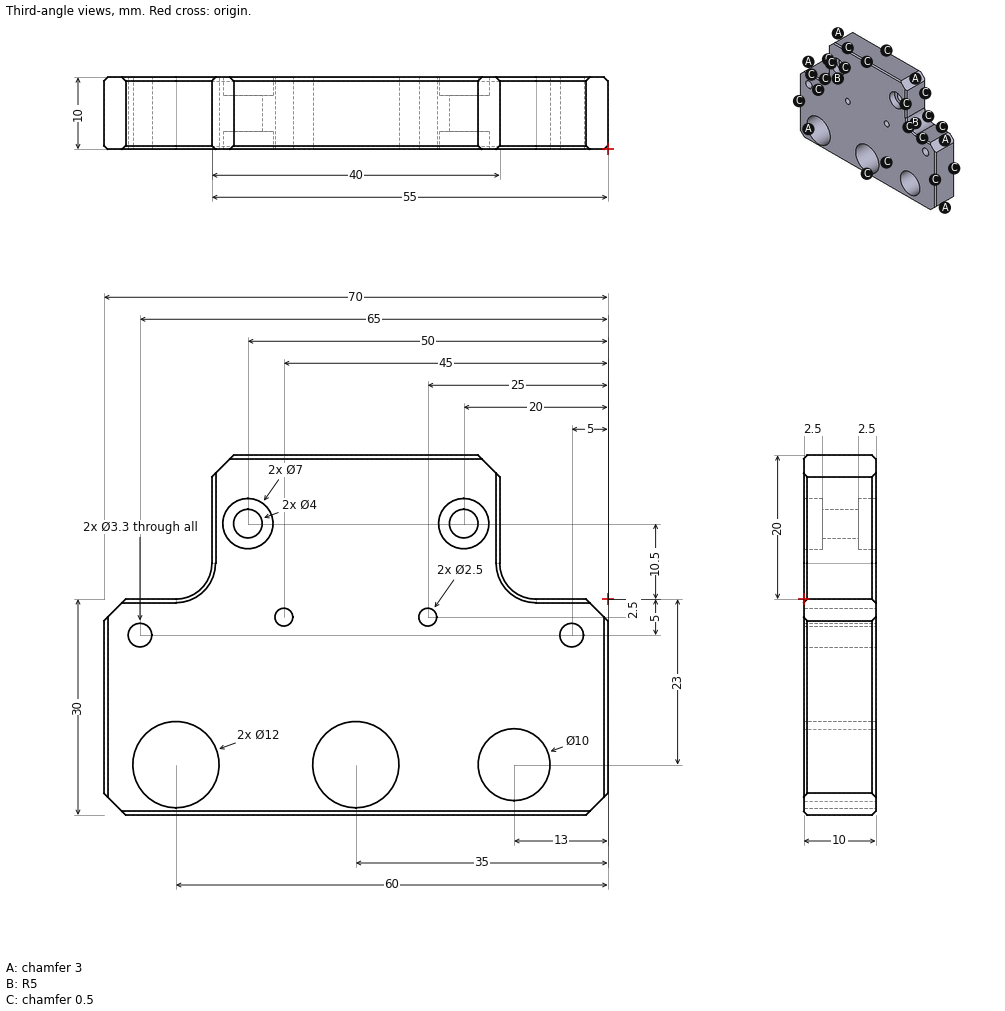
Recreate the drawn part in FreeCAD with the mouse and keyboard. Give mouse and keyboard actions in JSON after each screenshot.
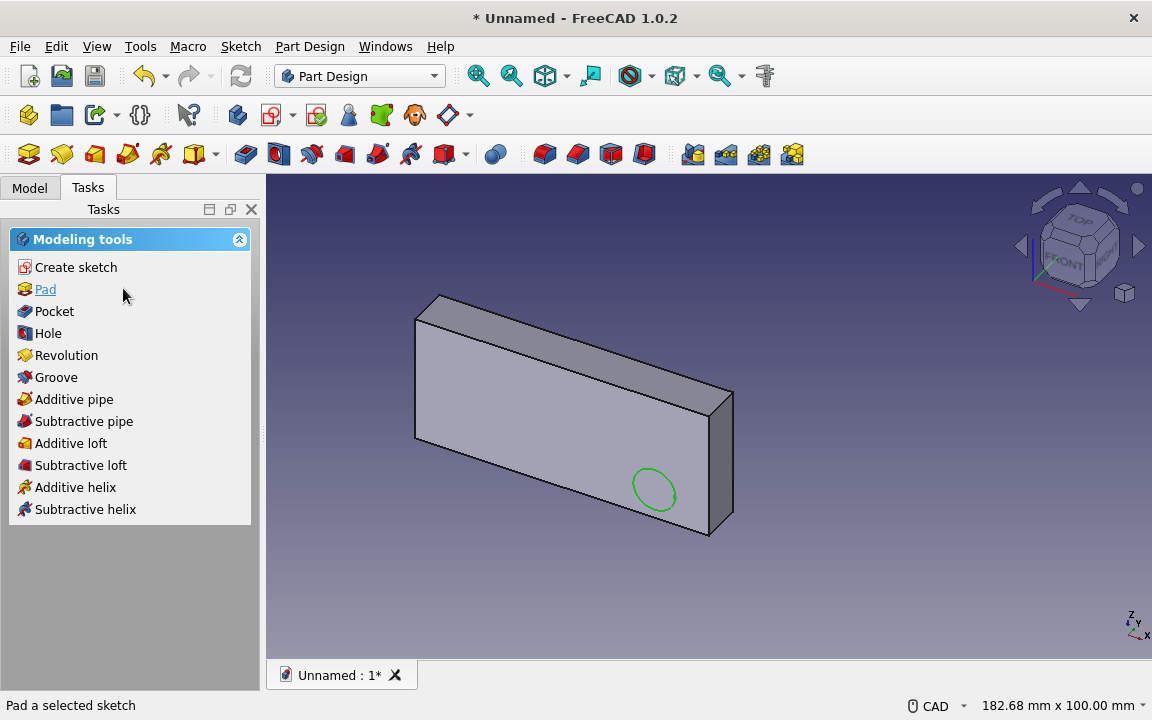
{"action": "left_click", "coordinate": [246, 154]}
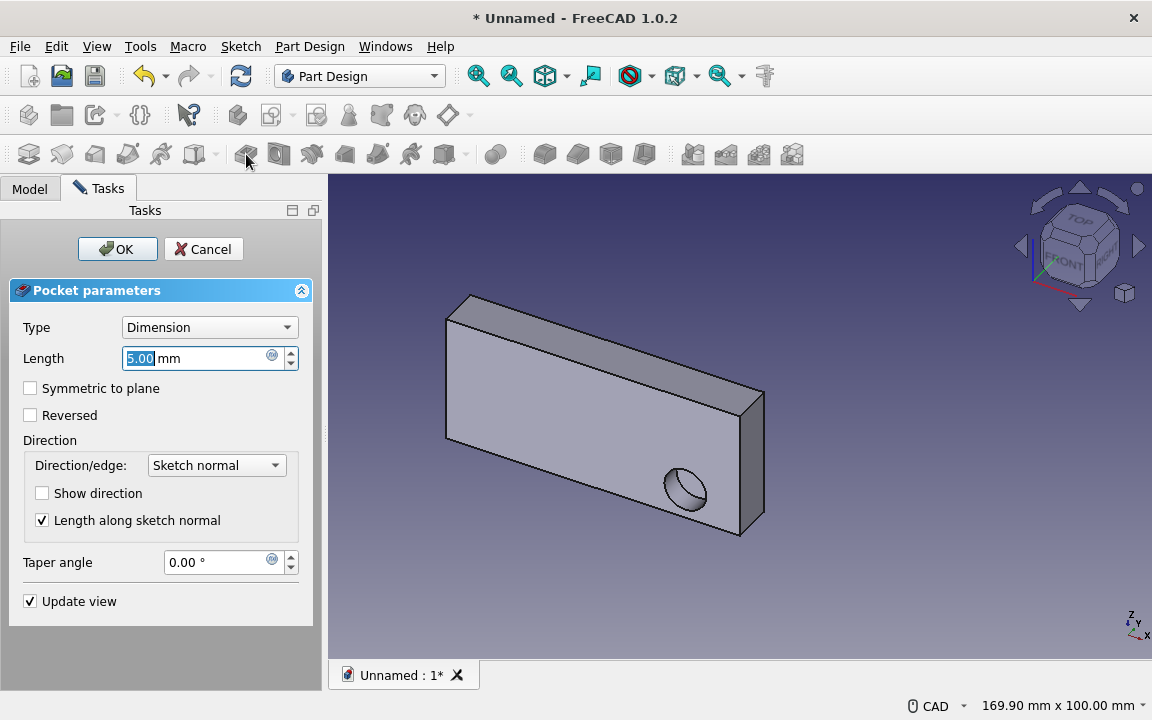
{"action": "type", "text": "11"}
{"action": "key", "text": "Tab"}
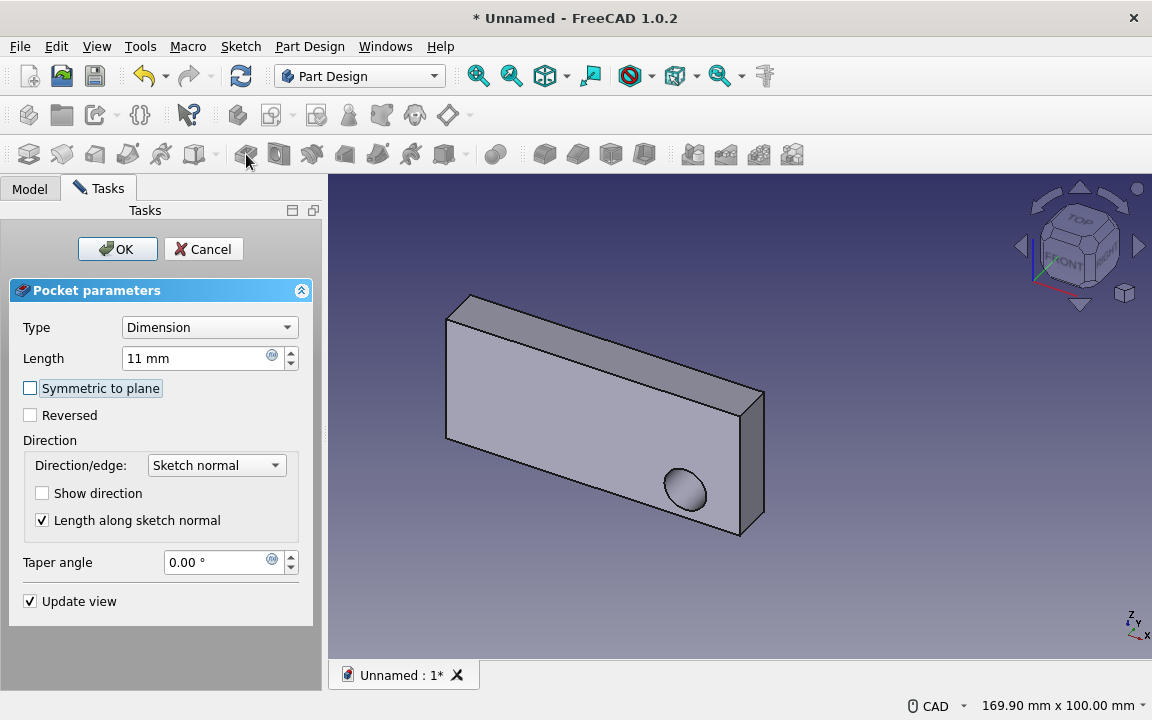
{"action": "left_click", "coordinate": [118, 249]}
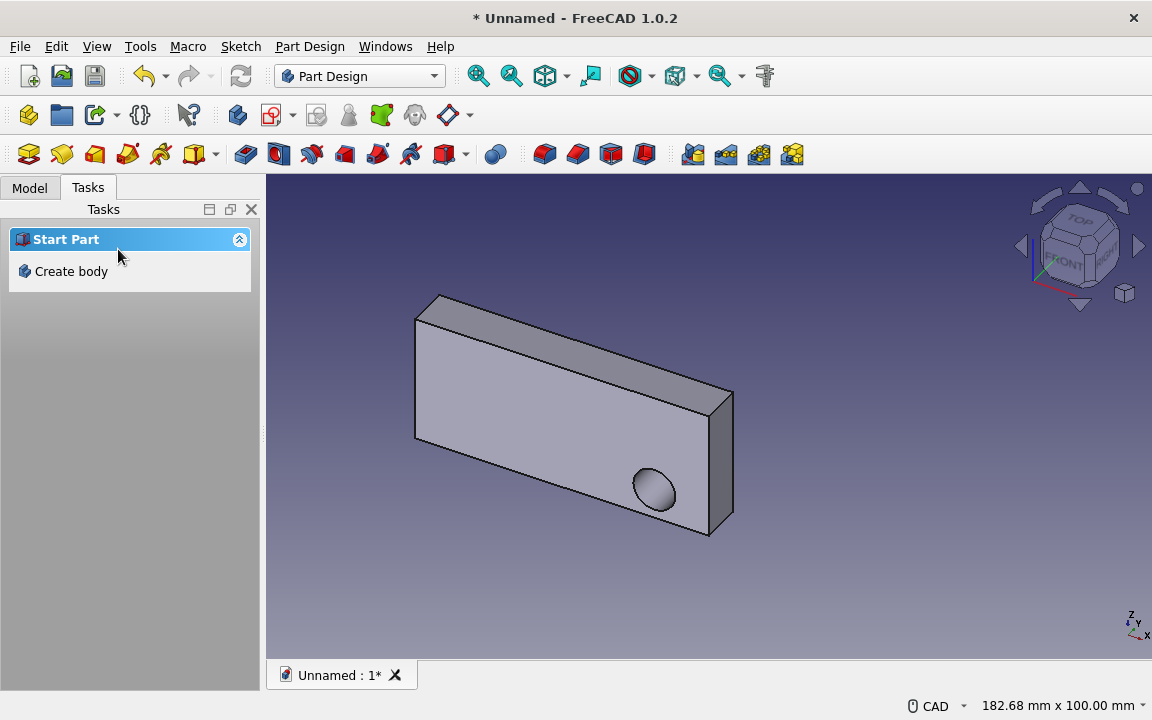
{"action": "left_click", "coordinate": [270, 116]}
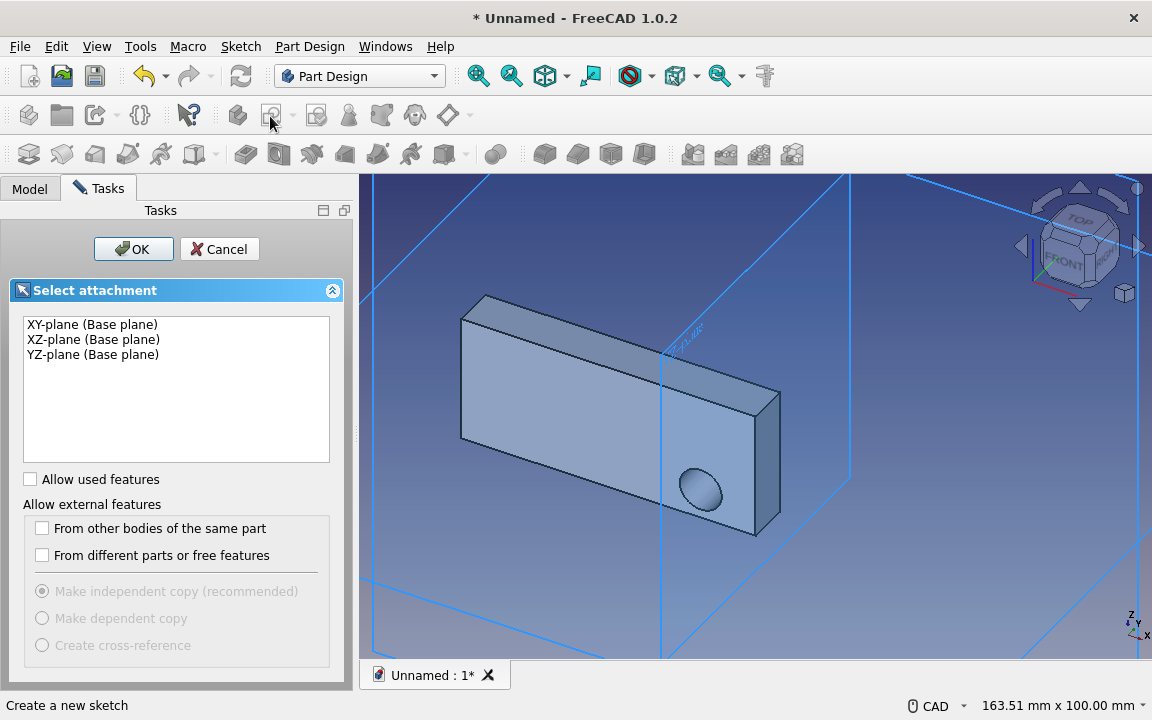
{"action": "left_click", "coordinate": [84, 340]}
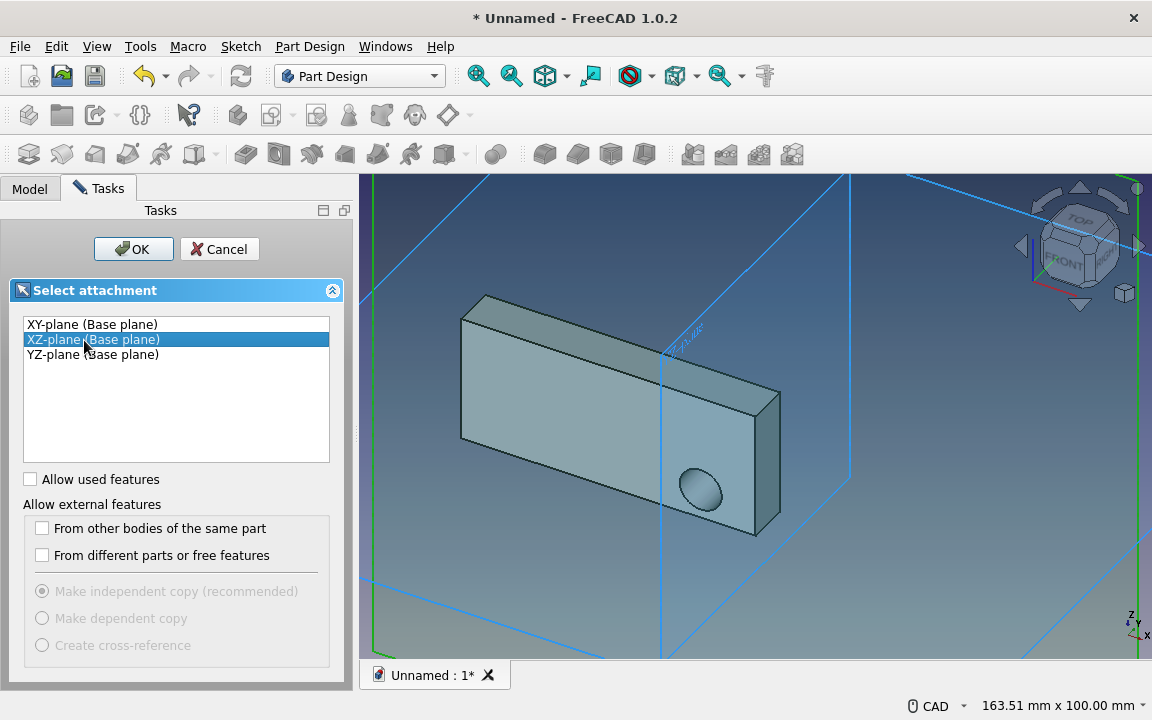
{"action": "left_click", "coordinate": [134, 249]}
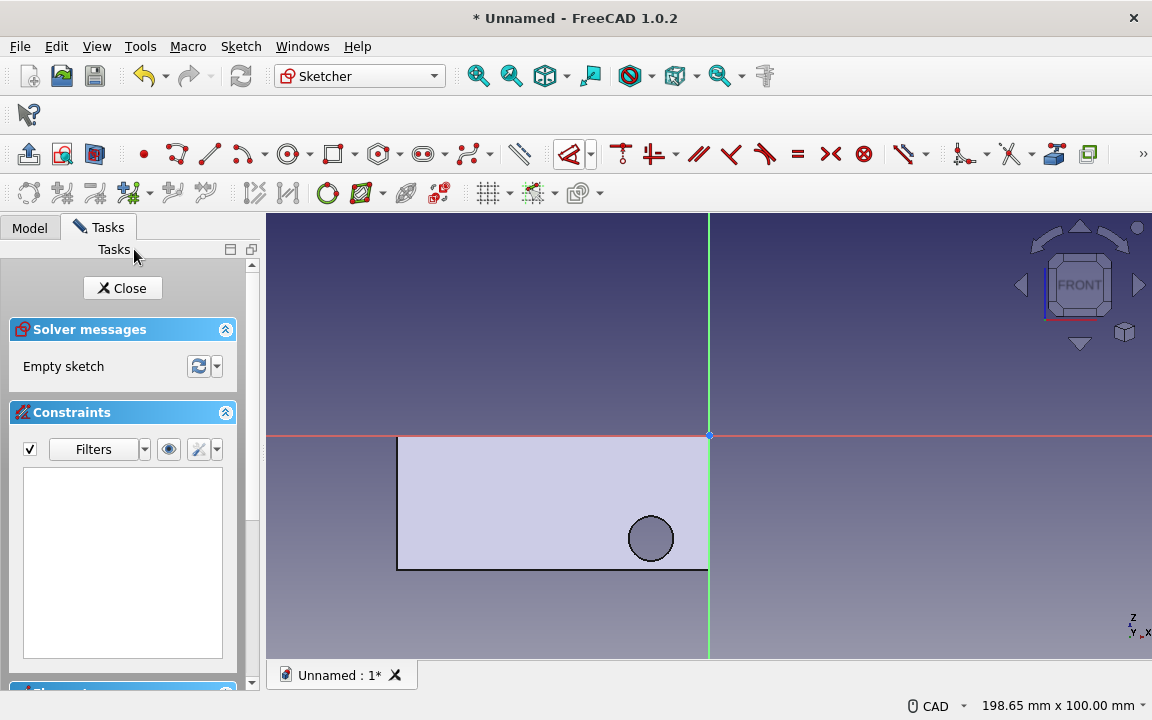
{"action": "scroll", "coordinate": [466, 579], "scroll_direction": "up", "scroll_amount": 3}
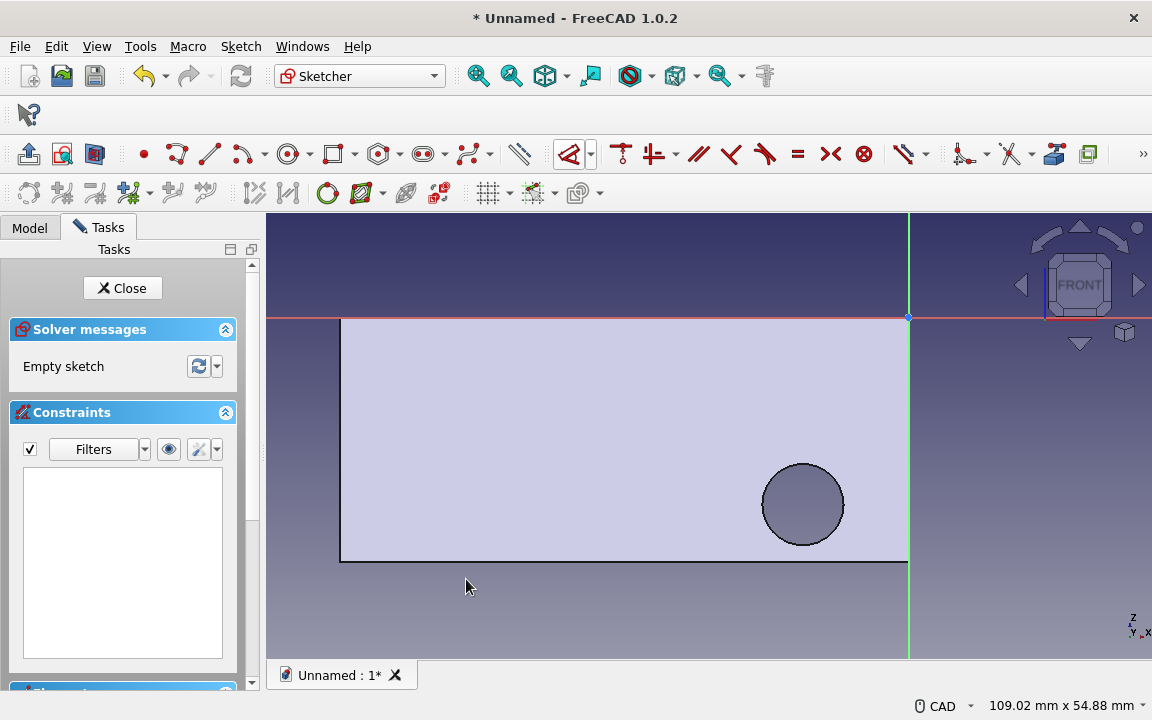
{"action": "left_click", "coordinate": [288, 154]}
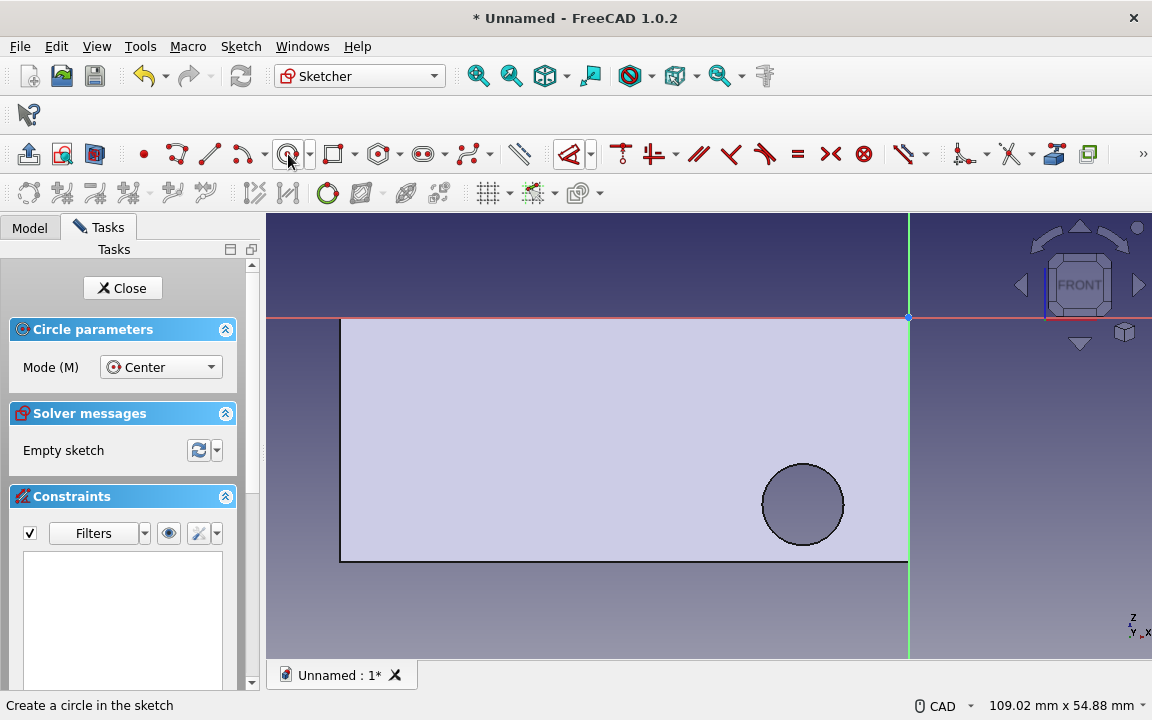
{"action": "left_click", "coordinate": [421, 505]}
{"action": "left_click", "coordinate": [455, 470]}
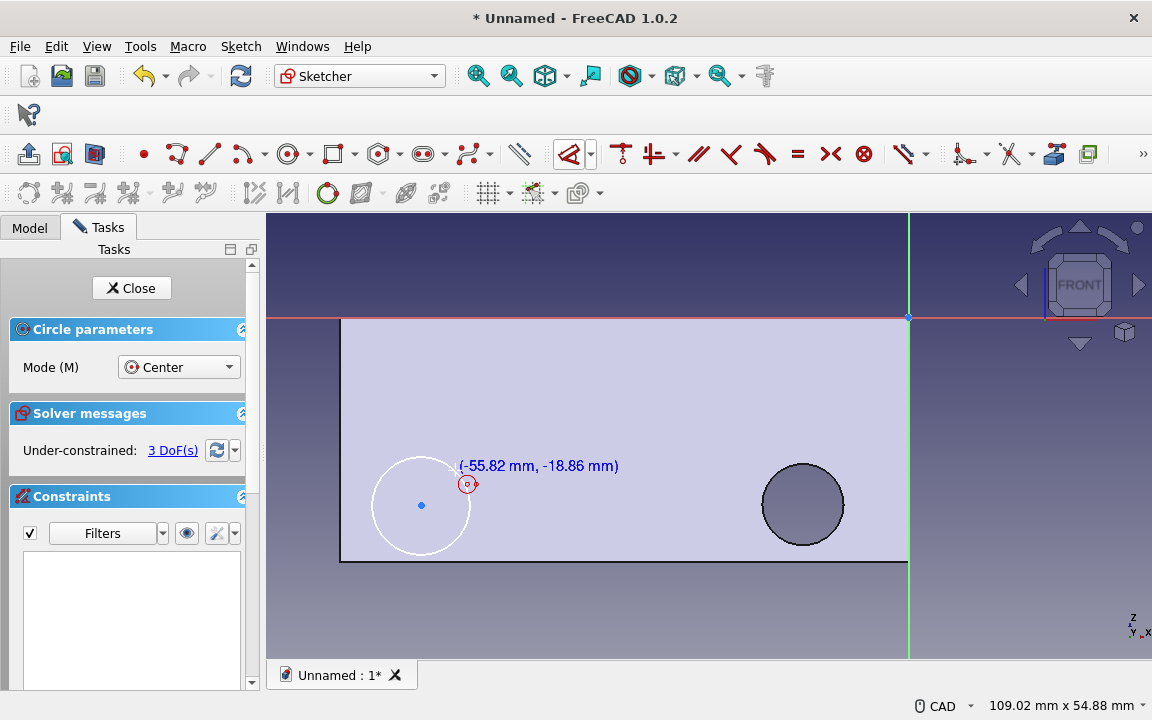
{"action": "left_click", "coordinate": [624, 505]}
{"action": "left_click", "coordinate": [659, 470]}
{"action": "key", "text": "Escape"}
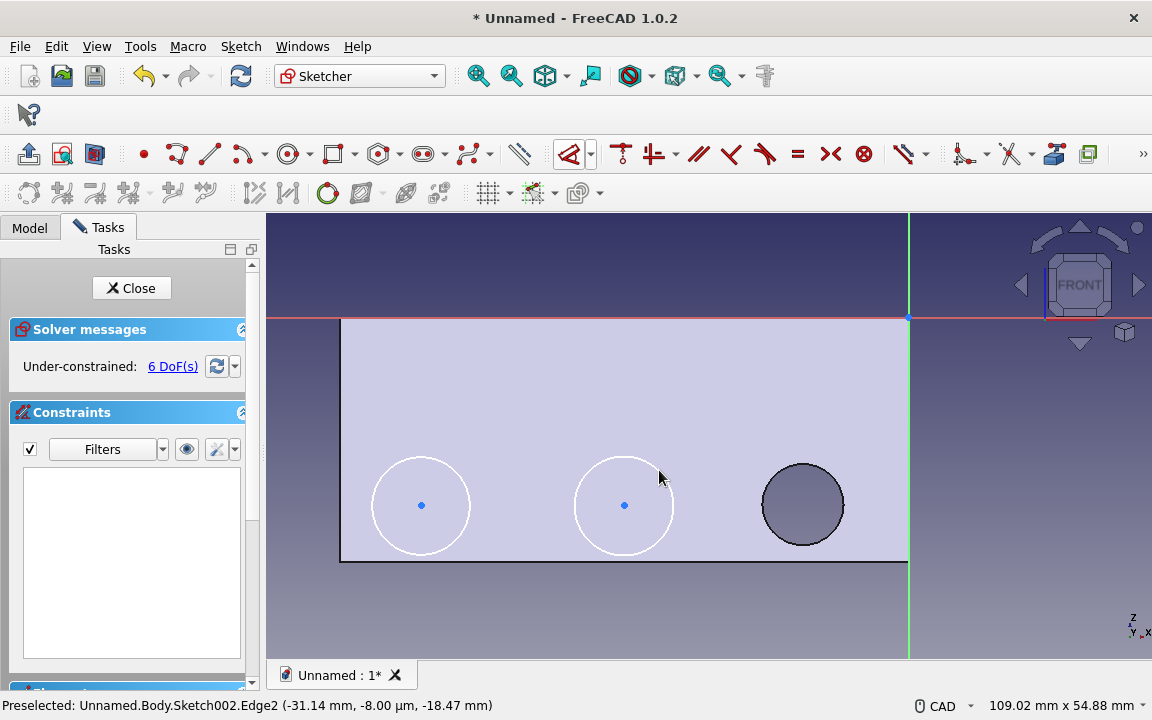
{"action": "left_click", "coordinate": [455, 471]}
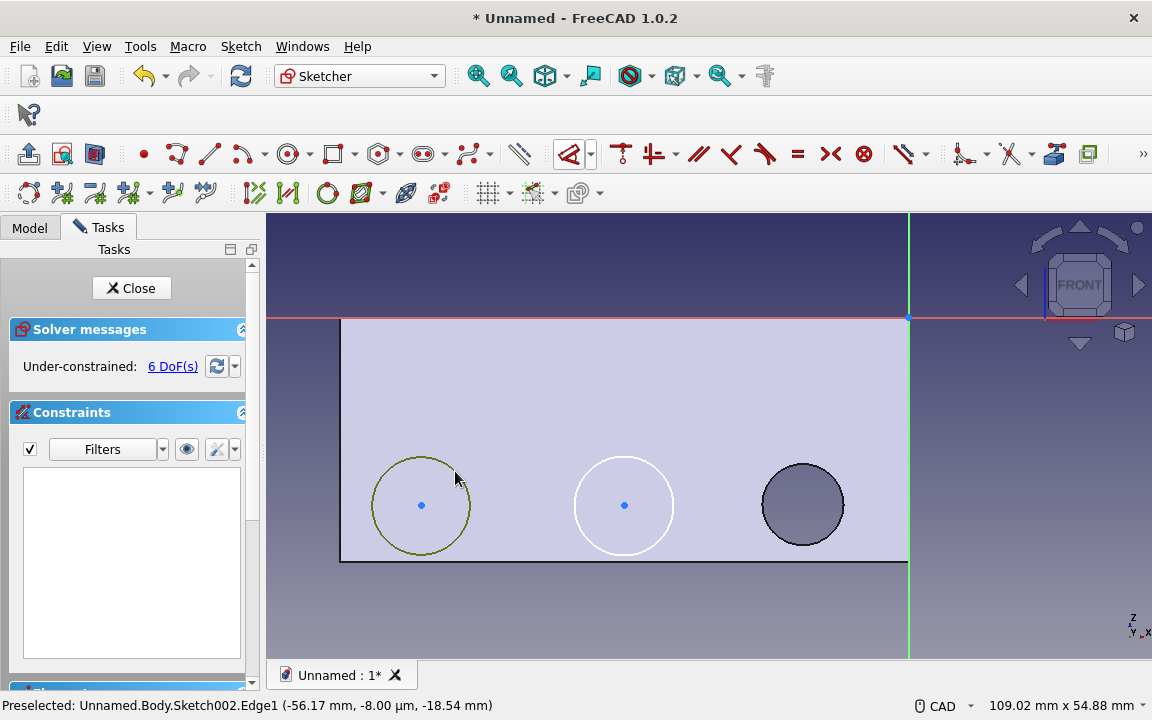
{"action": "left_click", "coordinate": [659, 471]}